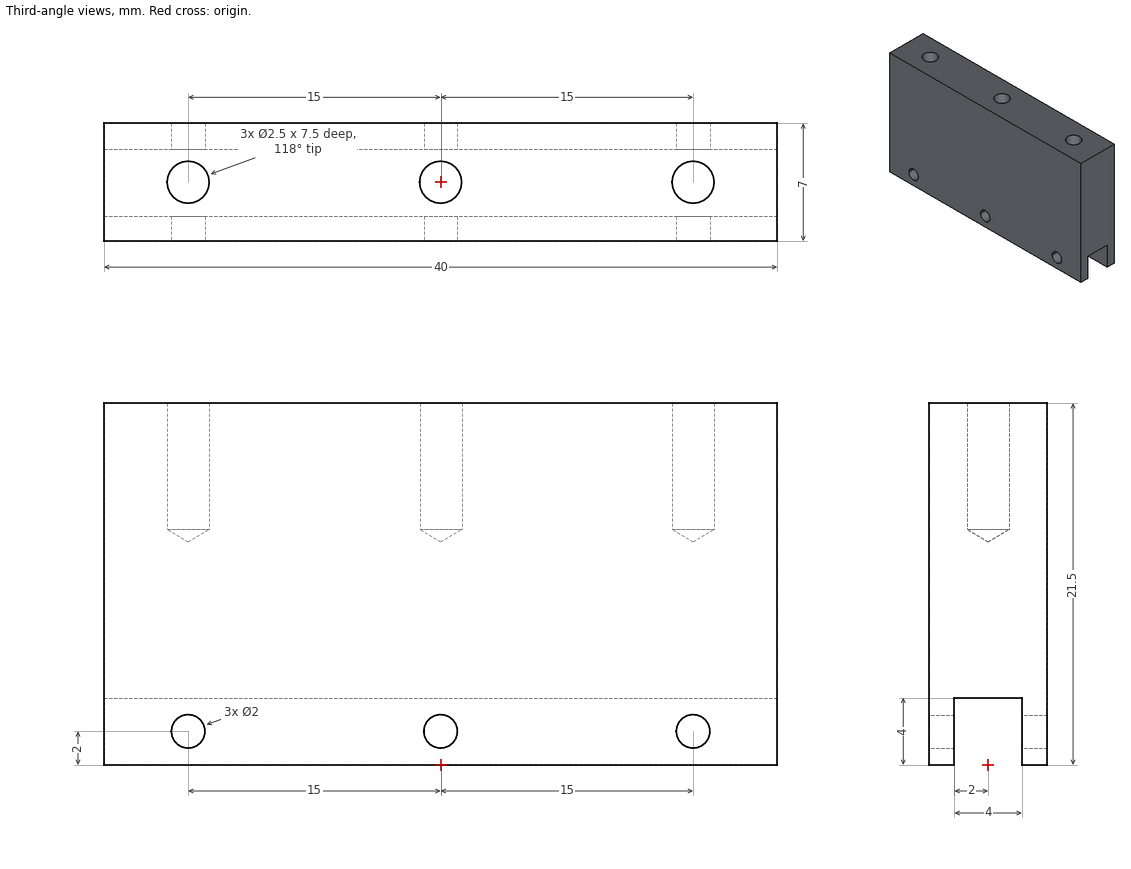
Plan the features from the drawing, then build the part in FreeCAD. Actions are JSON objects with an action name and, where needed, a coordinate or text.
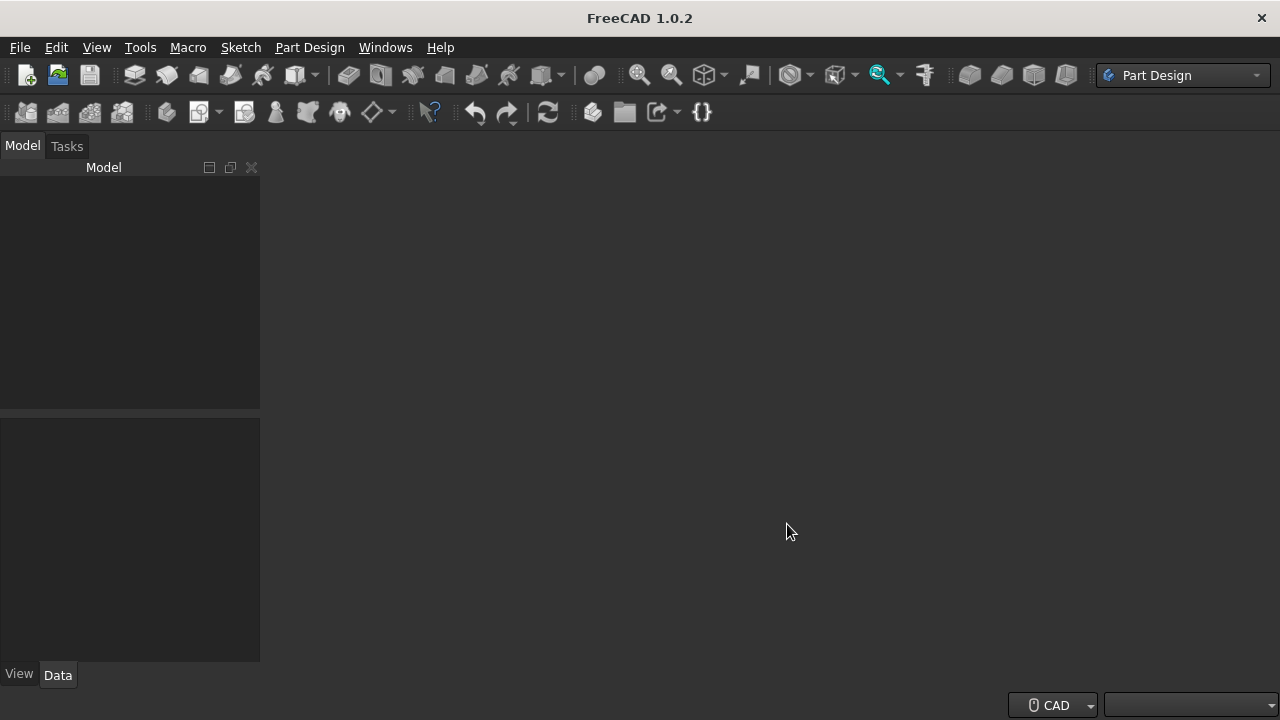
{"action": "left_click", "coordinate": [26, 76]}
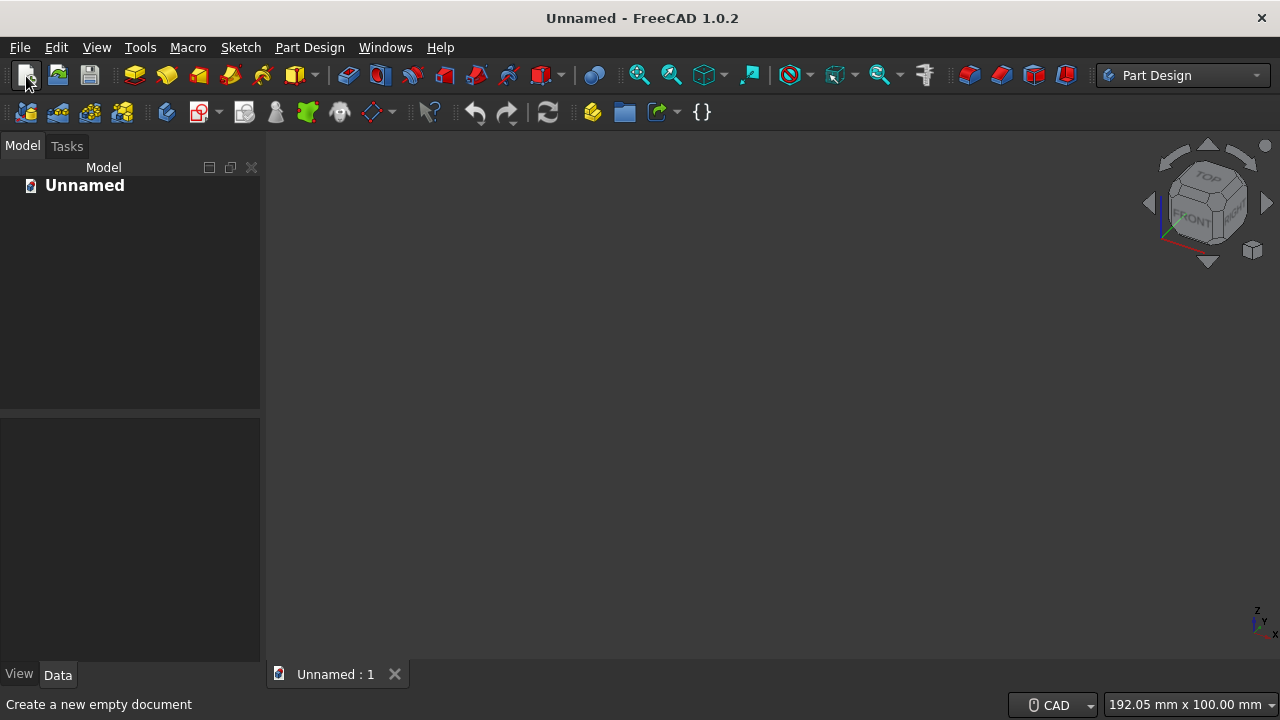
{"action": "left_click", "coordinate": [200, 112]}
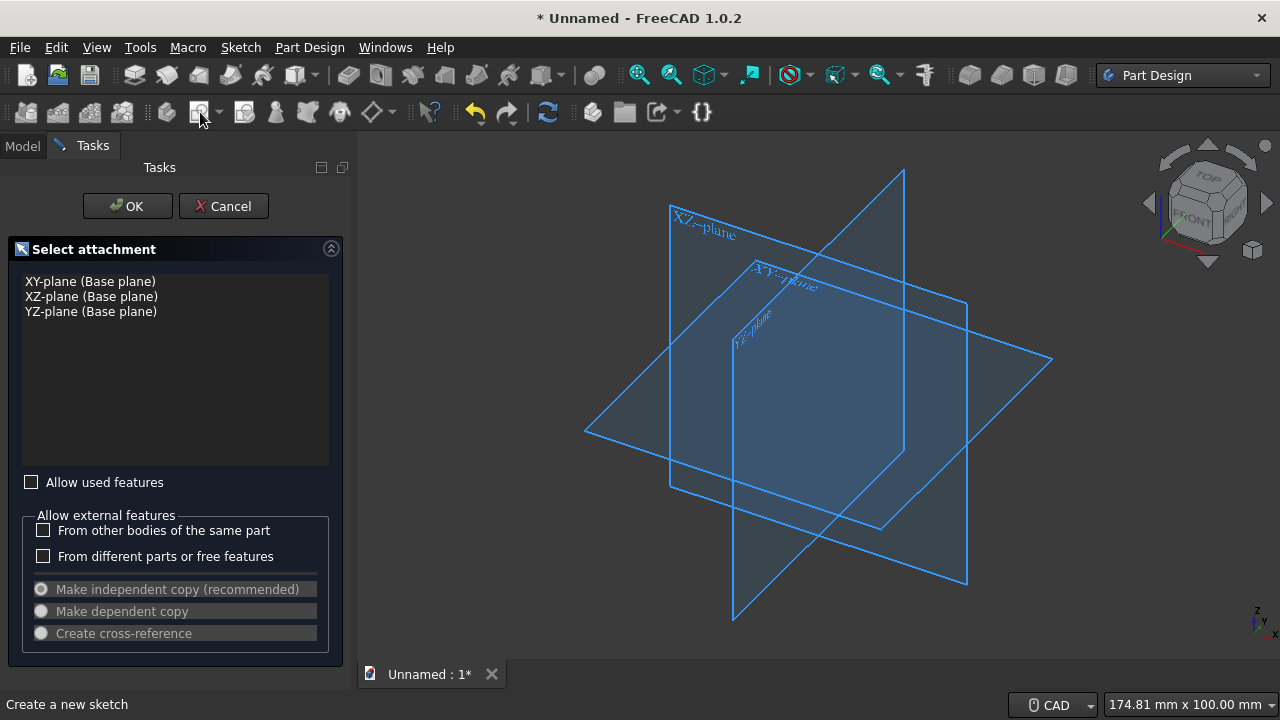
{"action": "left_click", "coordinate": [82, 282]}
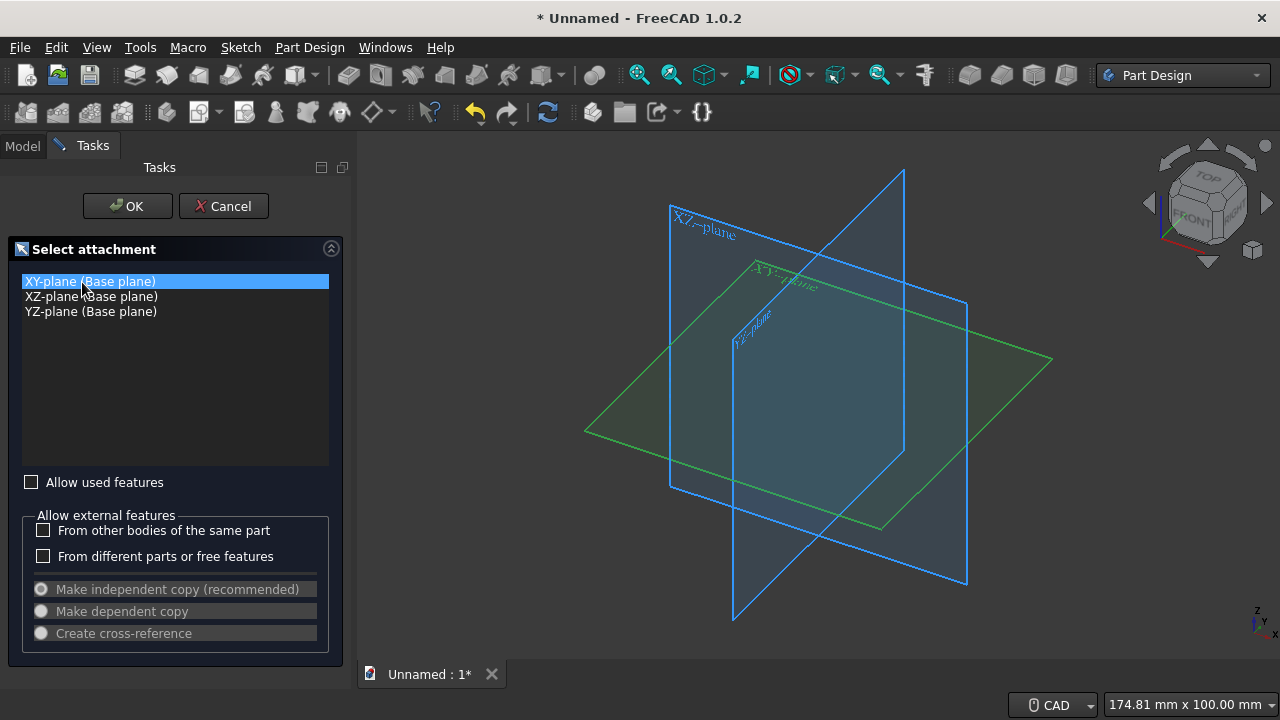
{"action": "left_click", "coordinate": [128, 206]}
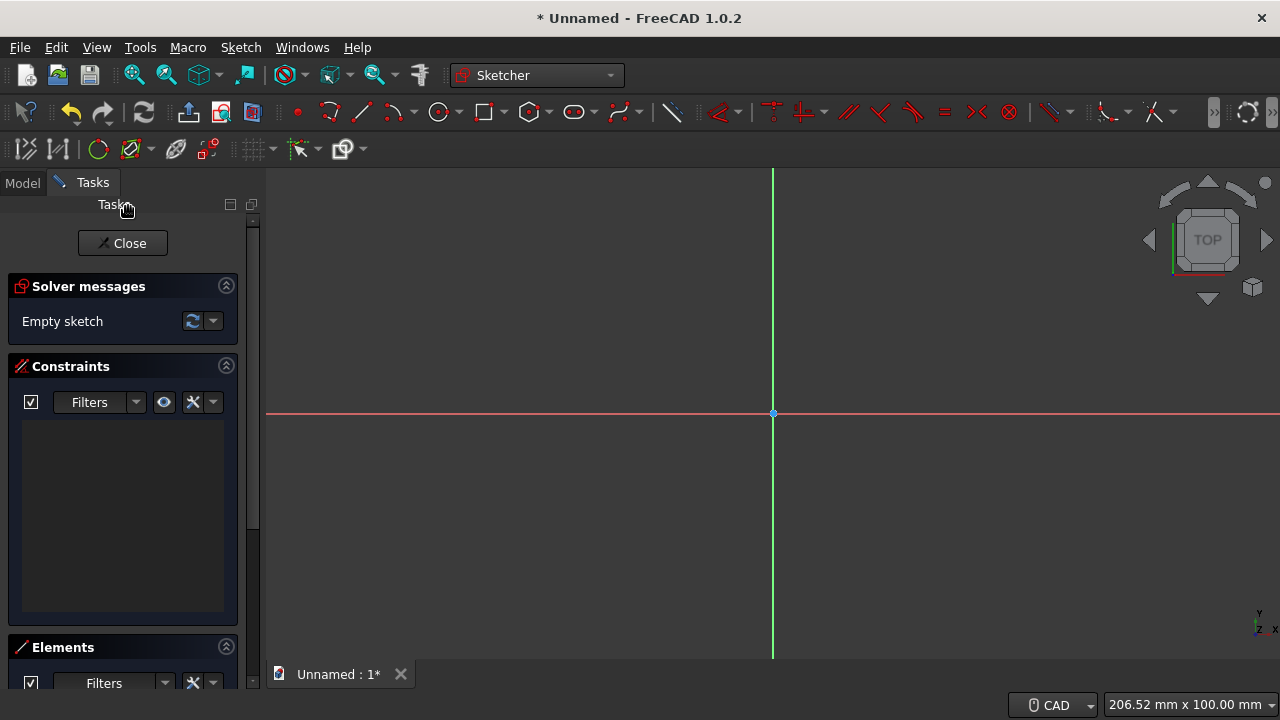
{"action": "scroll", "coordinate": [813, 414], "scroll_direction": "up", "scroll_amount": 5}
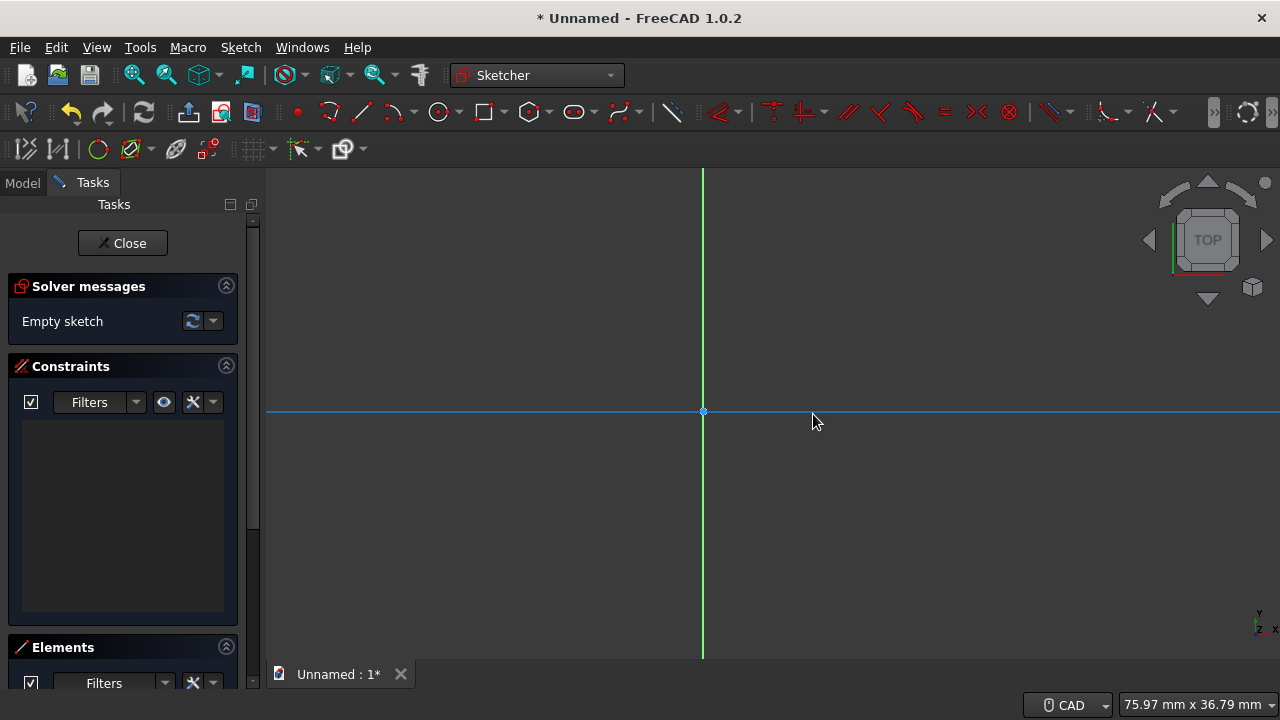
{"action": "key", "text": "g v"}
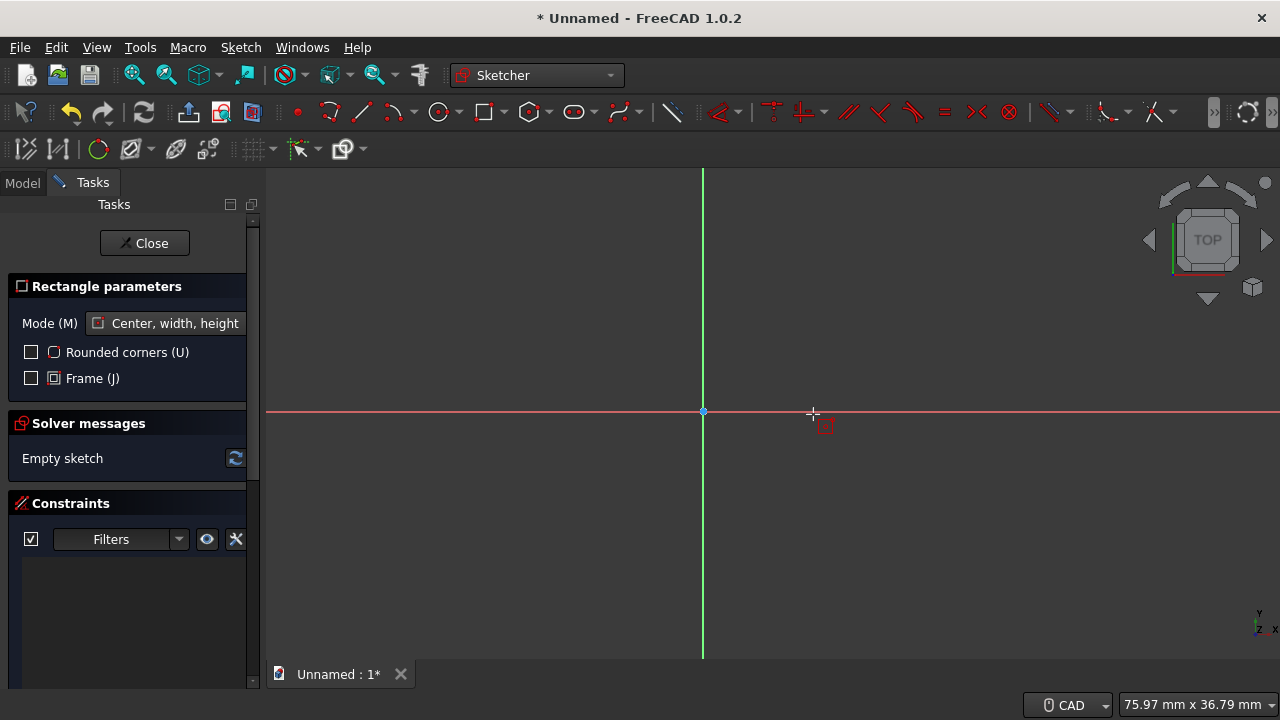
{"action": "left_click", "coordinate": [703, 412]}
{"action": "left_click", "coordinate": [970, 365]}
{"action": "key", "text": "Escape"}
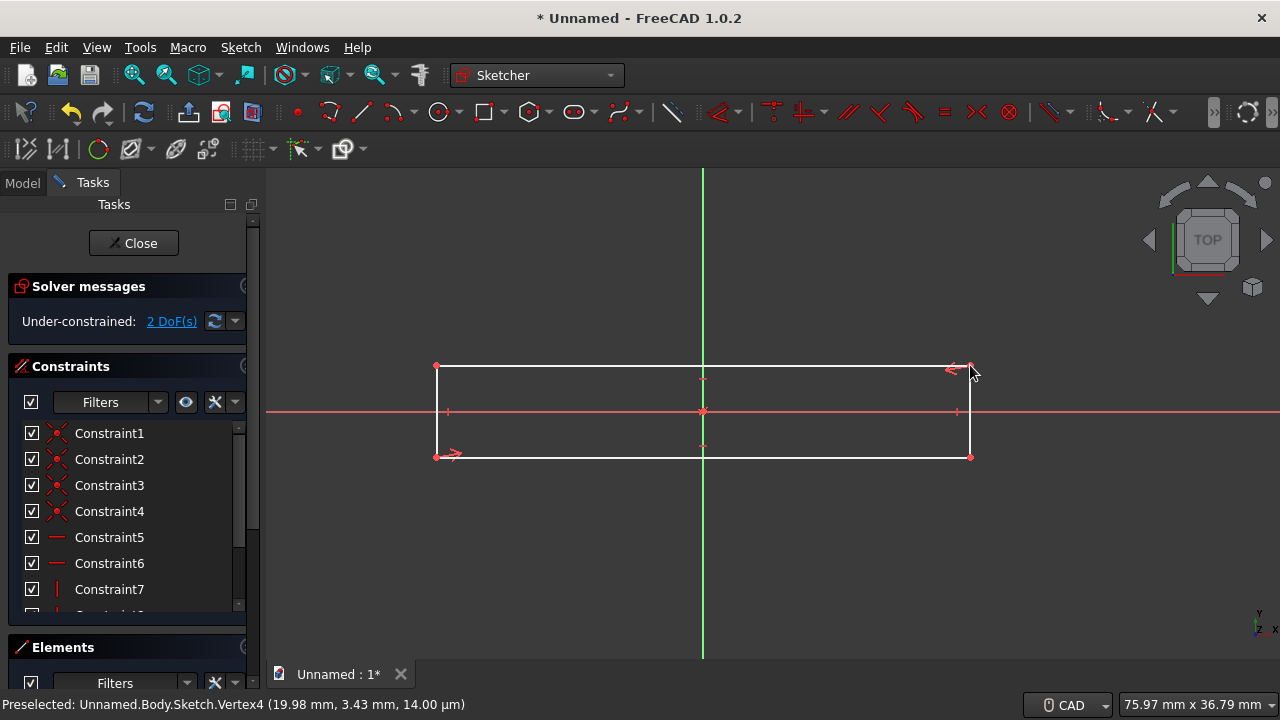
{"action": "left_click", "coordinate": [970, 430]}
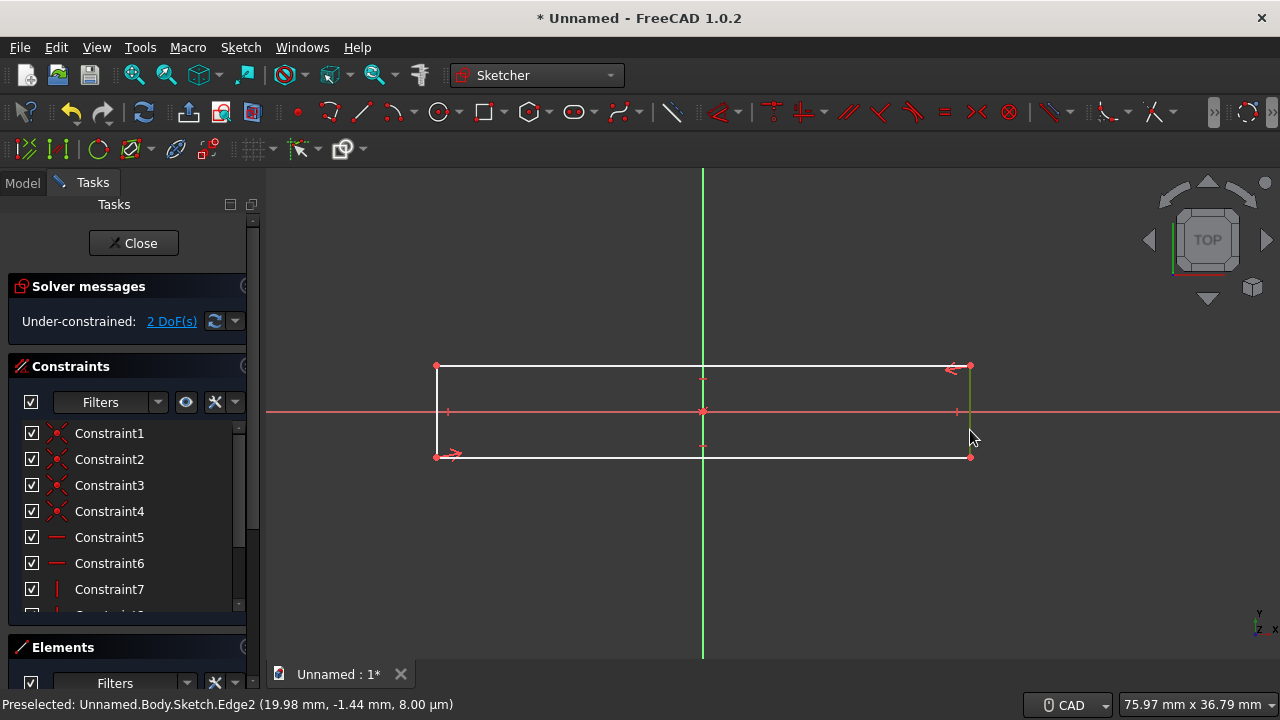
{"action": "left_click", "coordinate": [740, 112]}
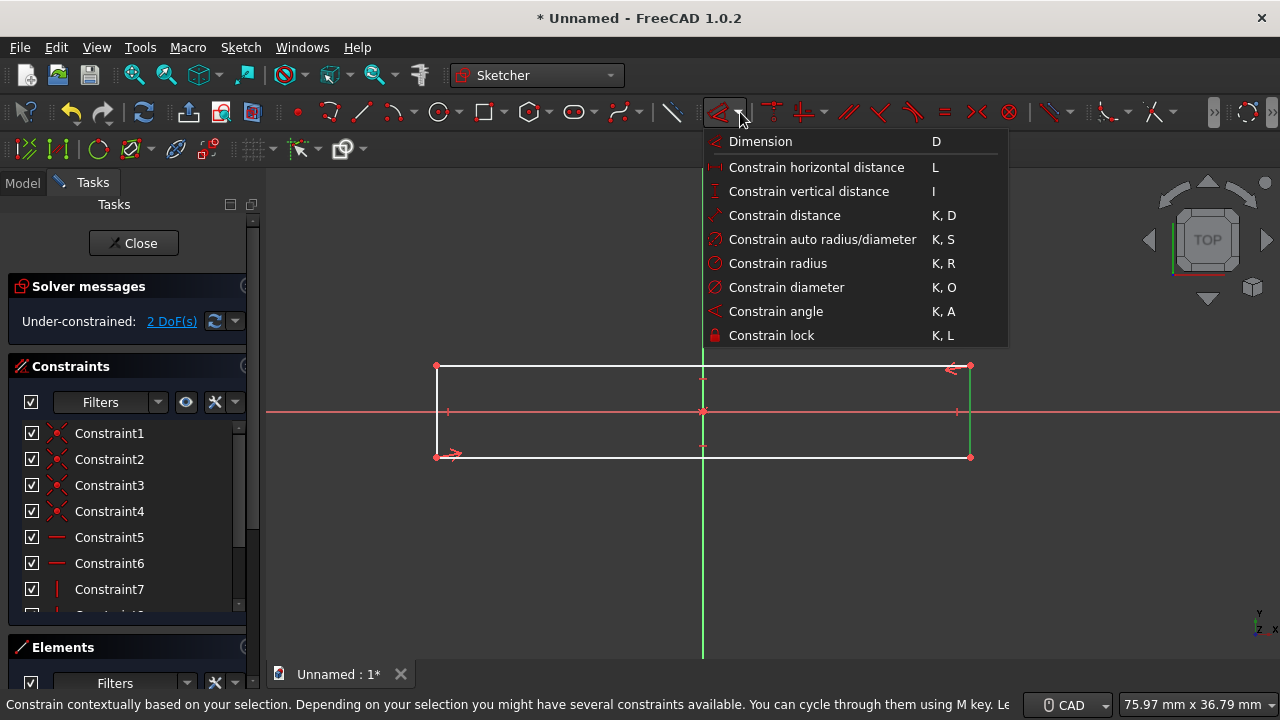
{"action": "left_click", "coordinate": [856, 191]}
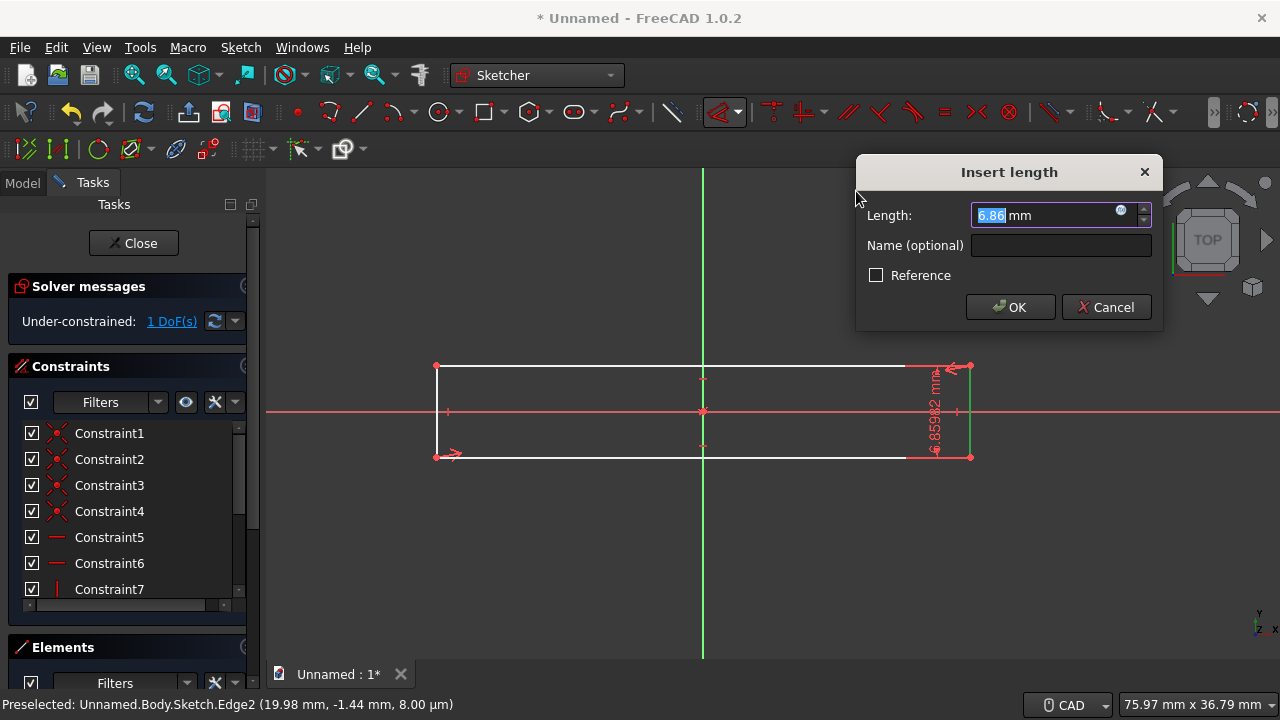
{"action": "type", "text": "7"}
{"action": "key", "text": "Return"}